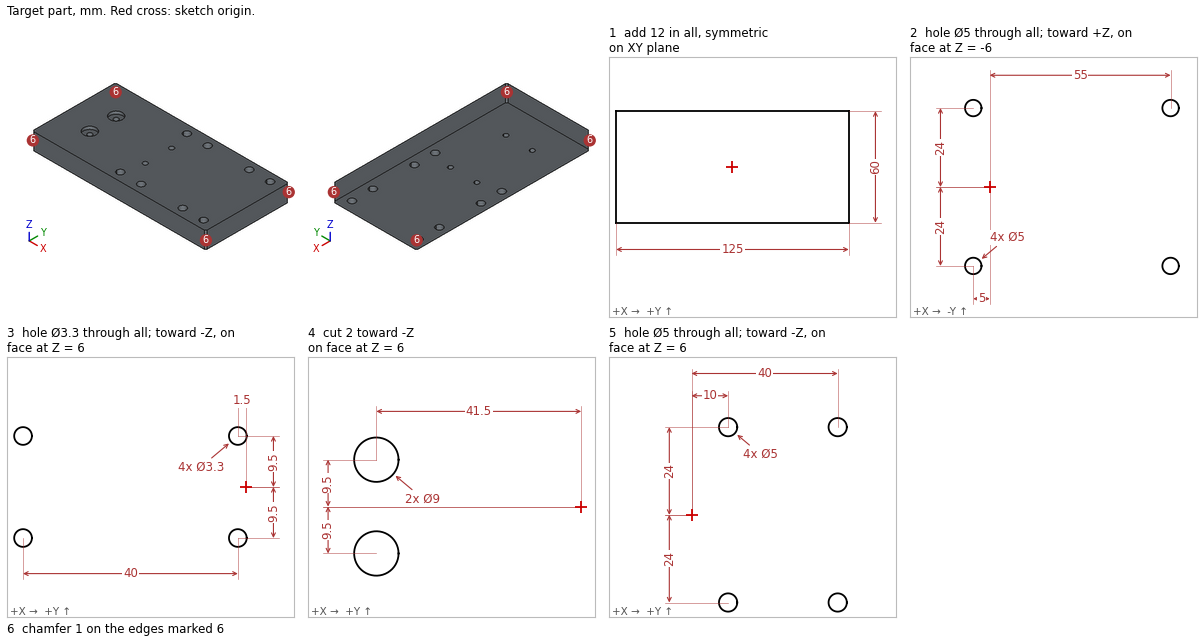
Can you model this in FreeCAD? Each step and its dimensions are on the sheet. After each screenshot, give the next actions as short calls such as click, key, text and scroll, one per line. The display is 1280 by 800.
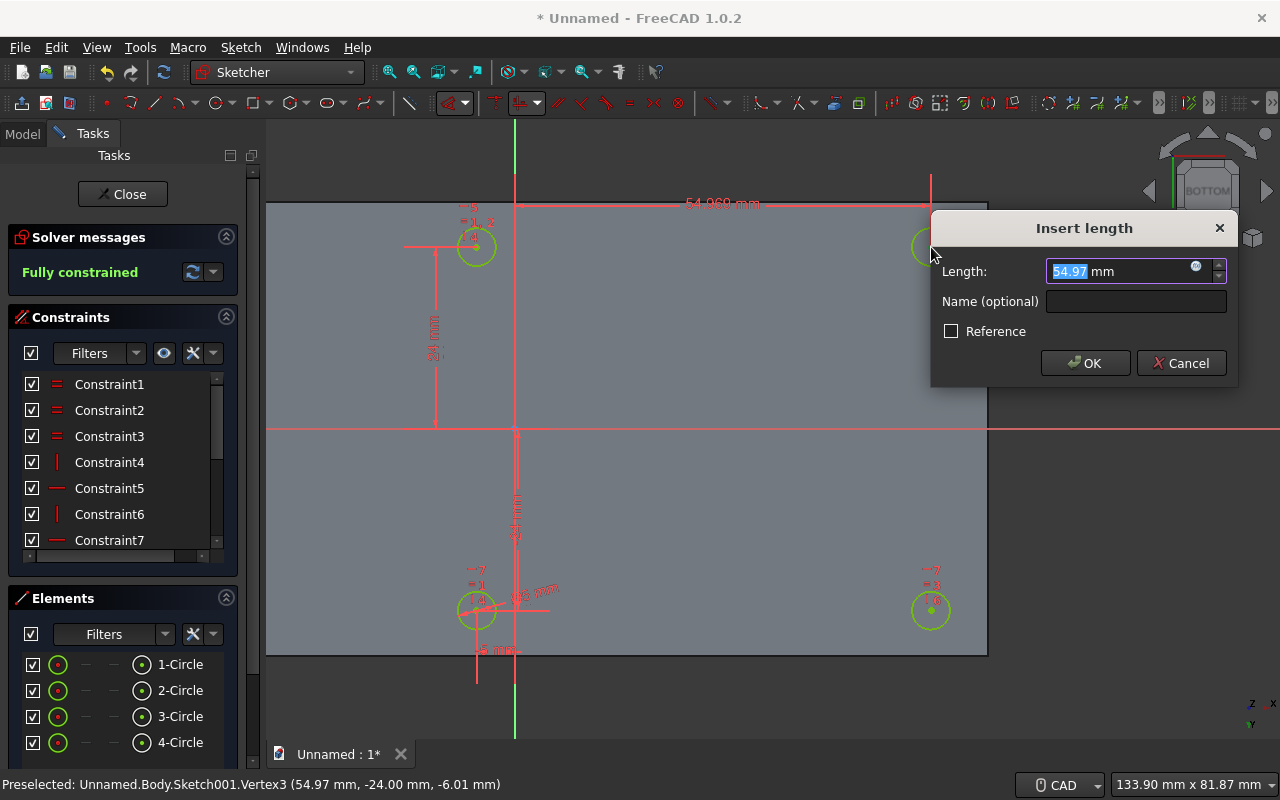
text(55)
key(Return)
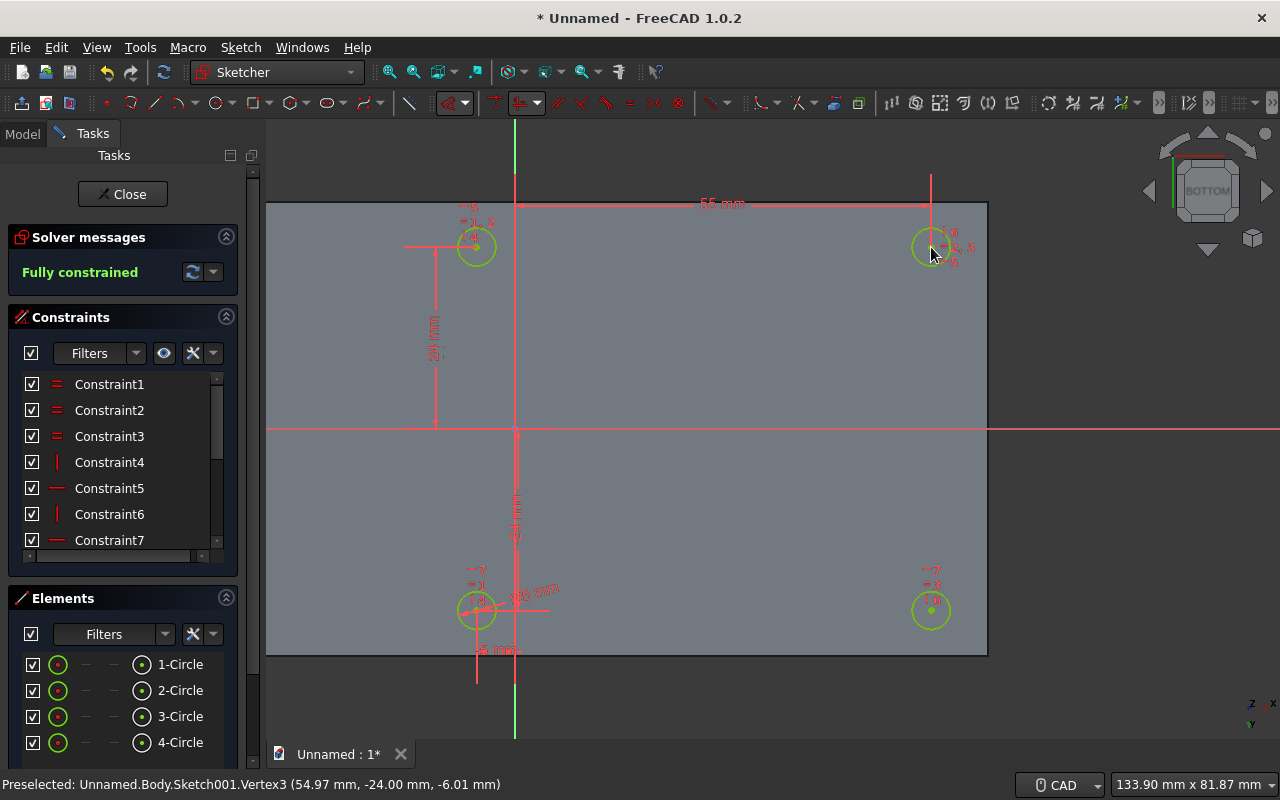
click(123, 194)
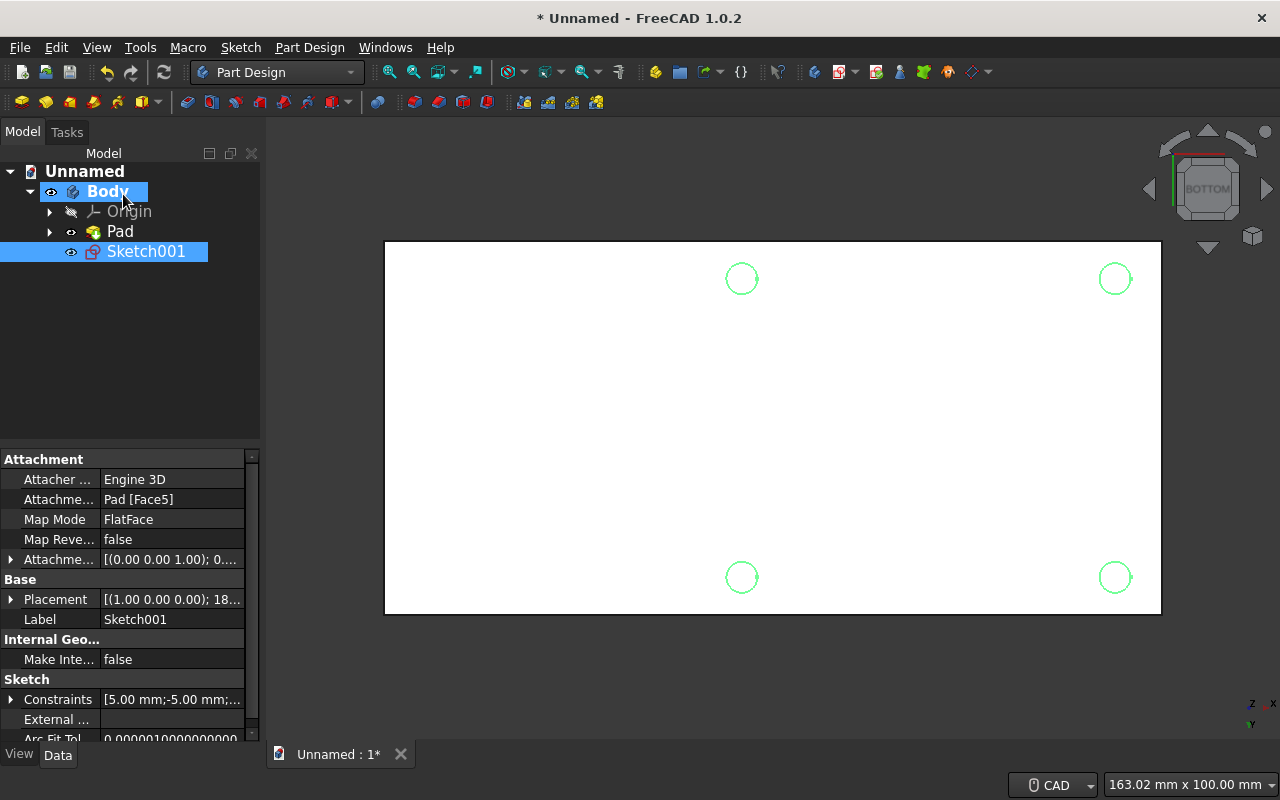
click(212, 102)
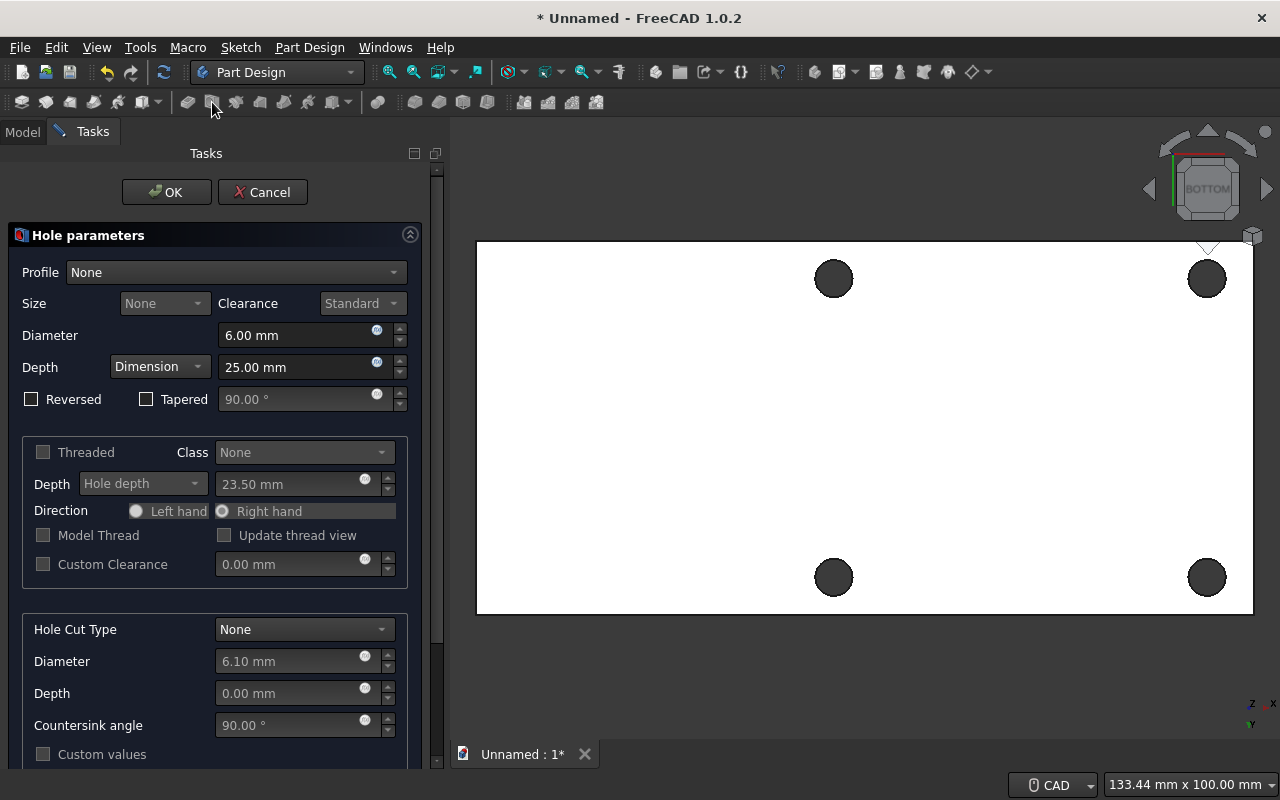
triple_click(305, 335)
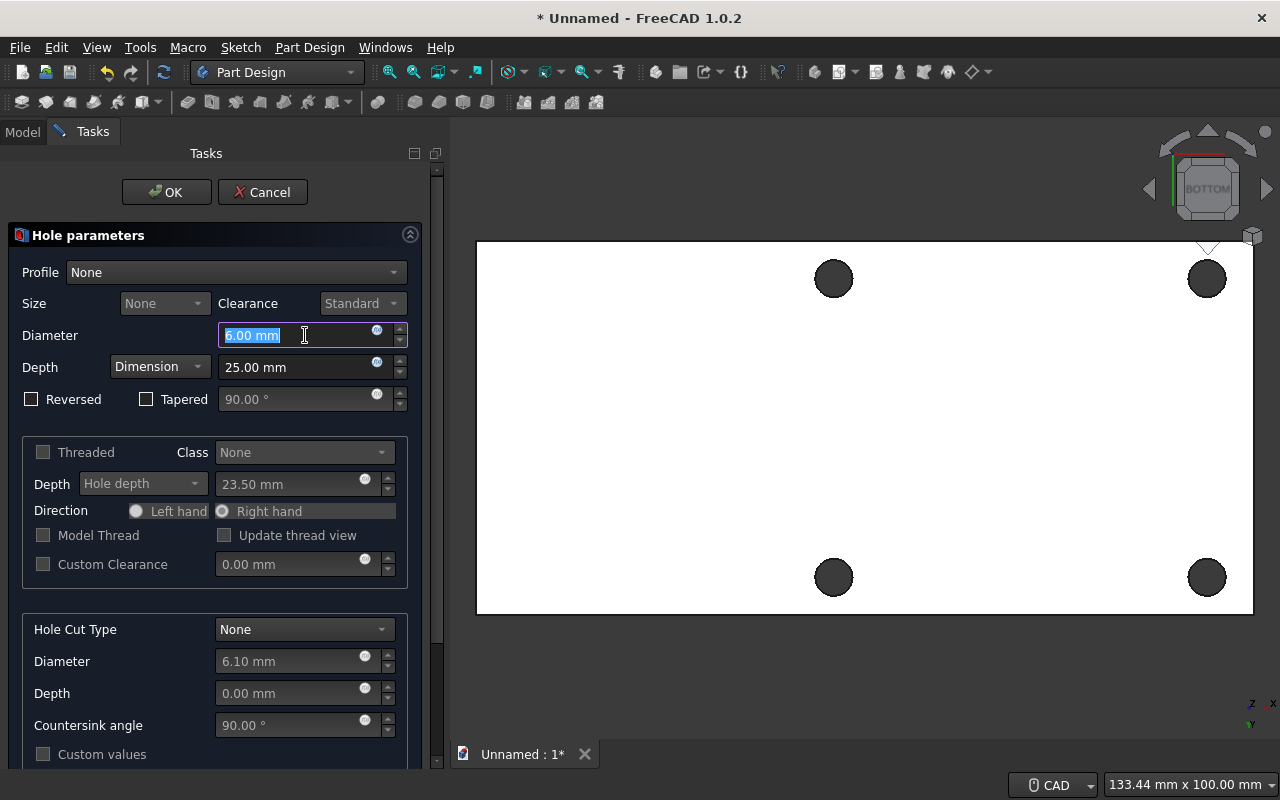
text(5)
key(Tab)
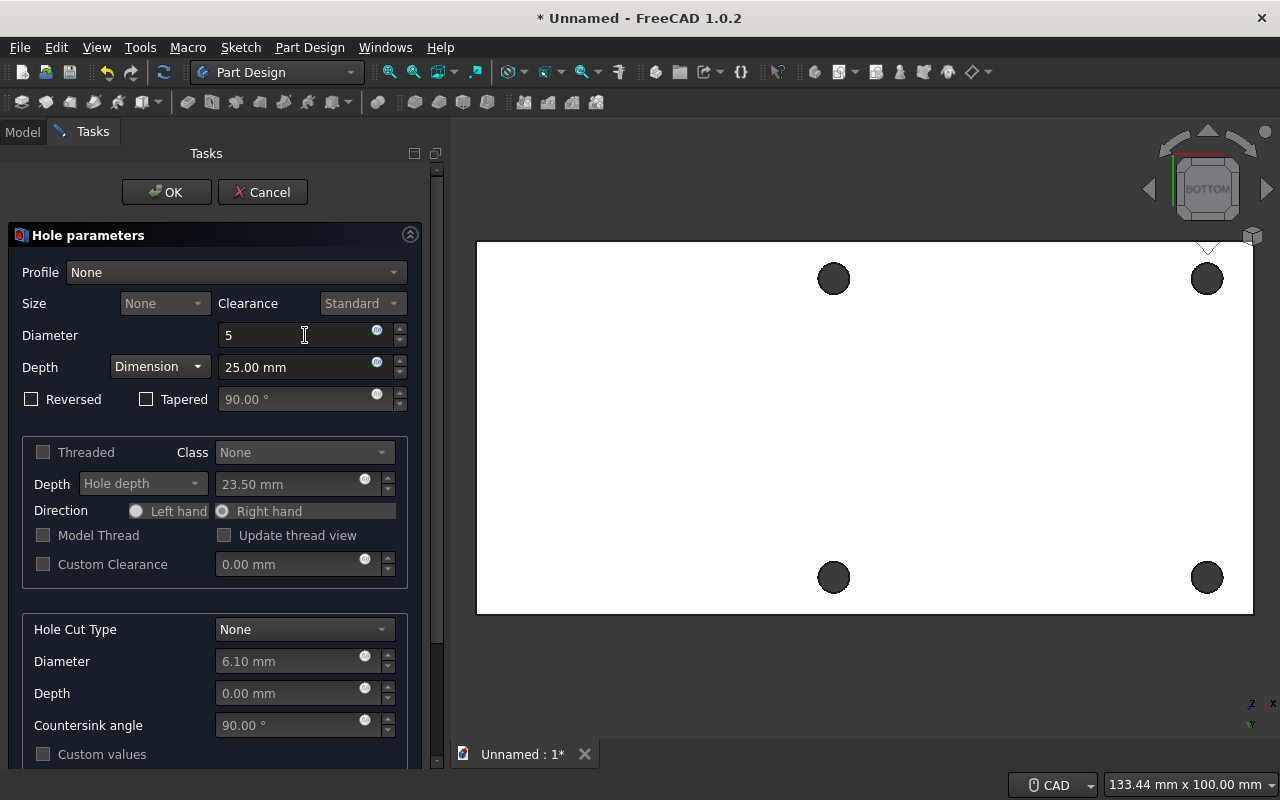
click(161, 366)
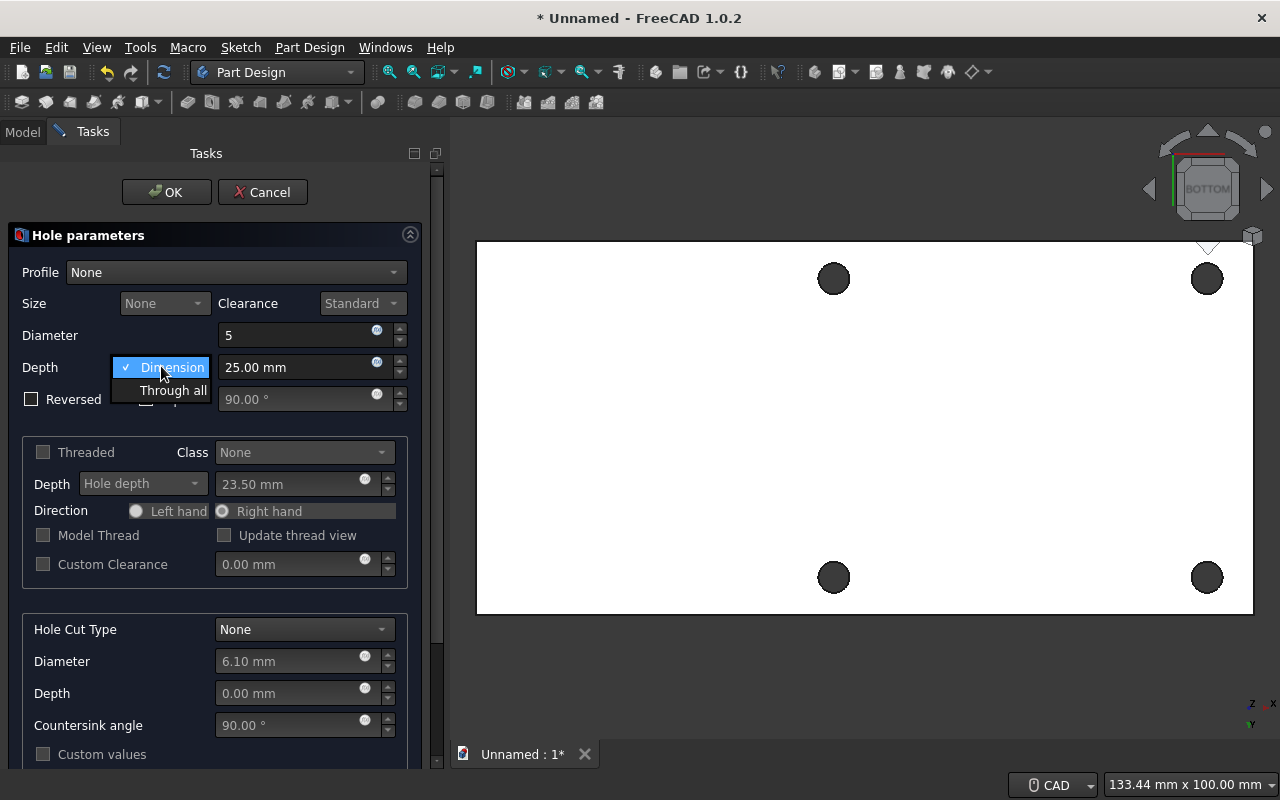
click(160, 390)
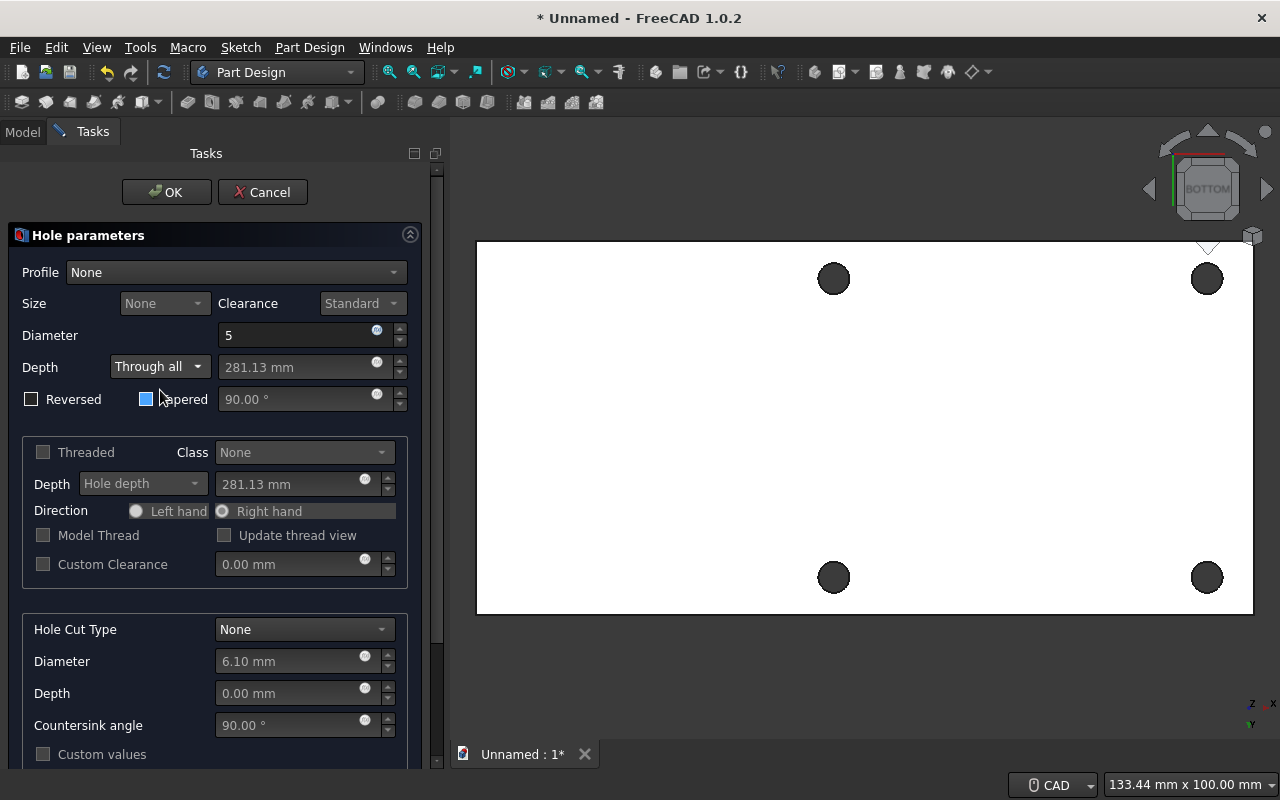
click(167, 192)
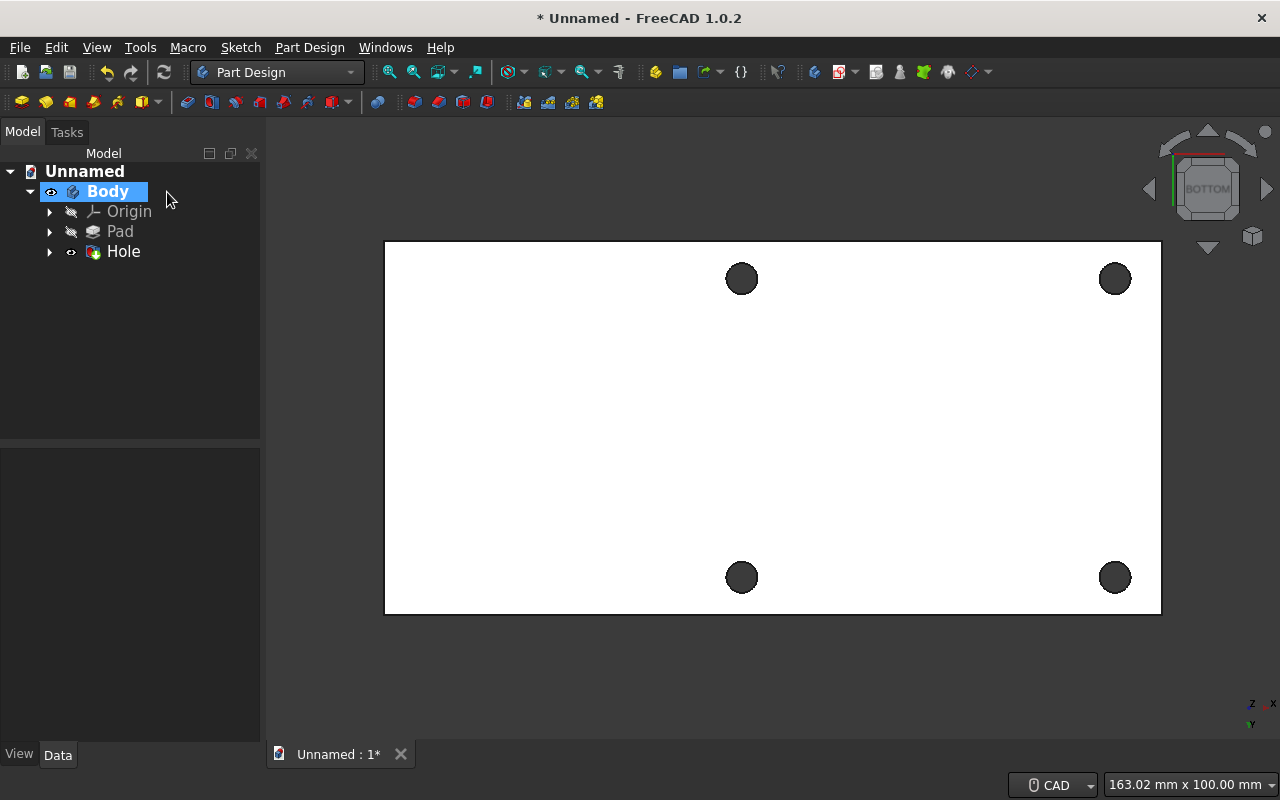
key(0)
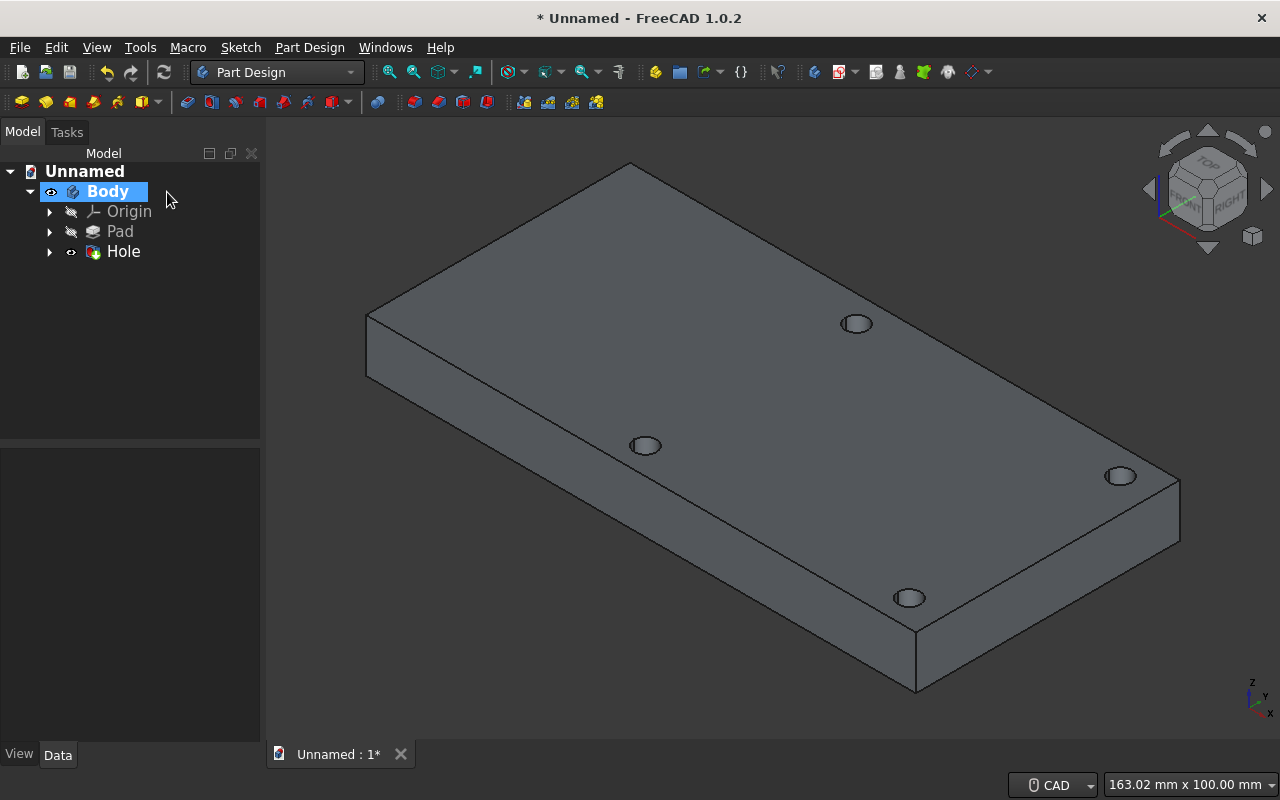
click(852, 442)